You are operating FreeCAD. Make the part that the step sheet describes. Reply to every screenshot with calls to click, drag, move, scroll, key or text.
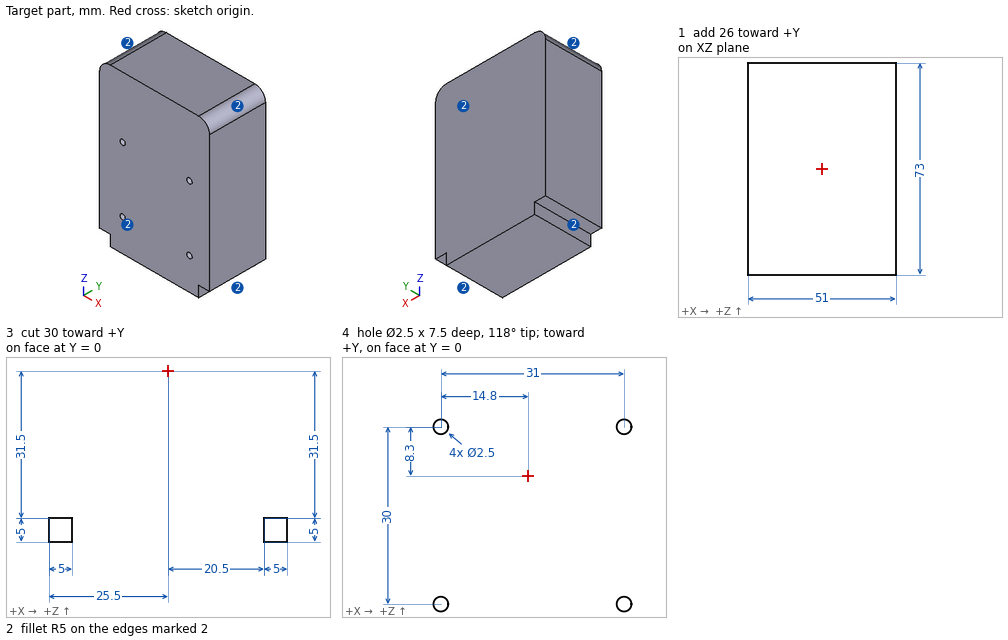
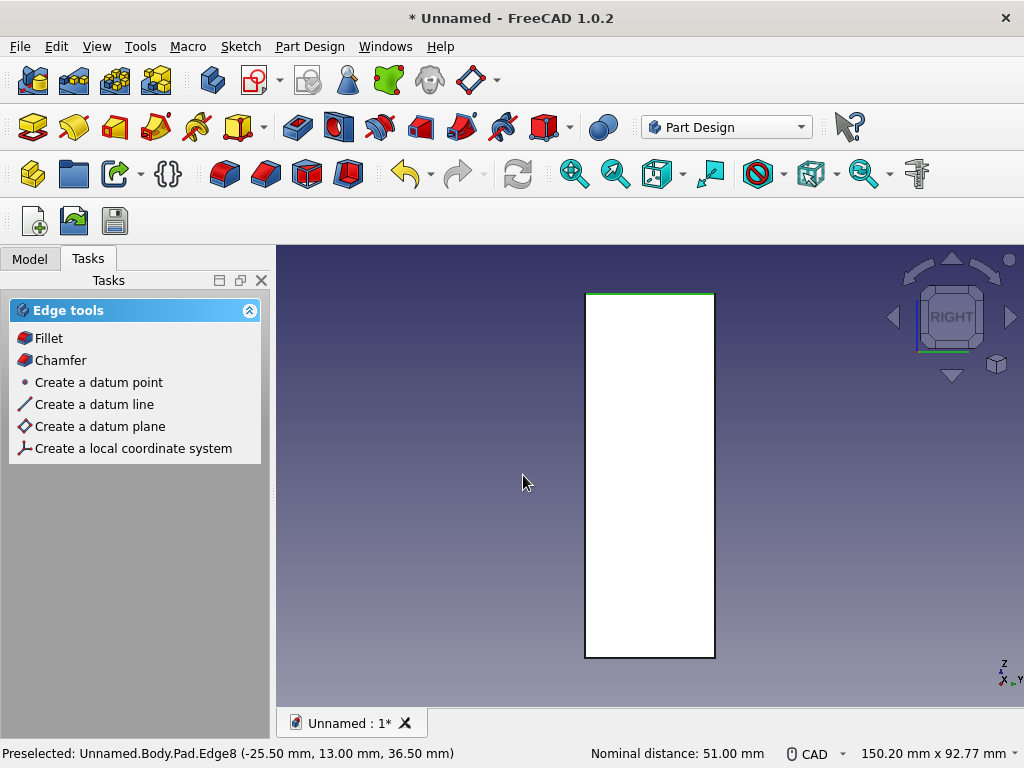
click(650, 657, ctrl)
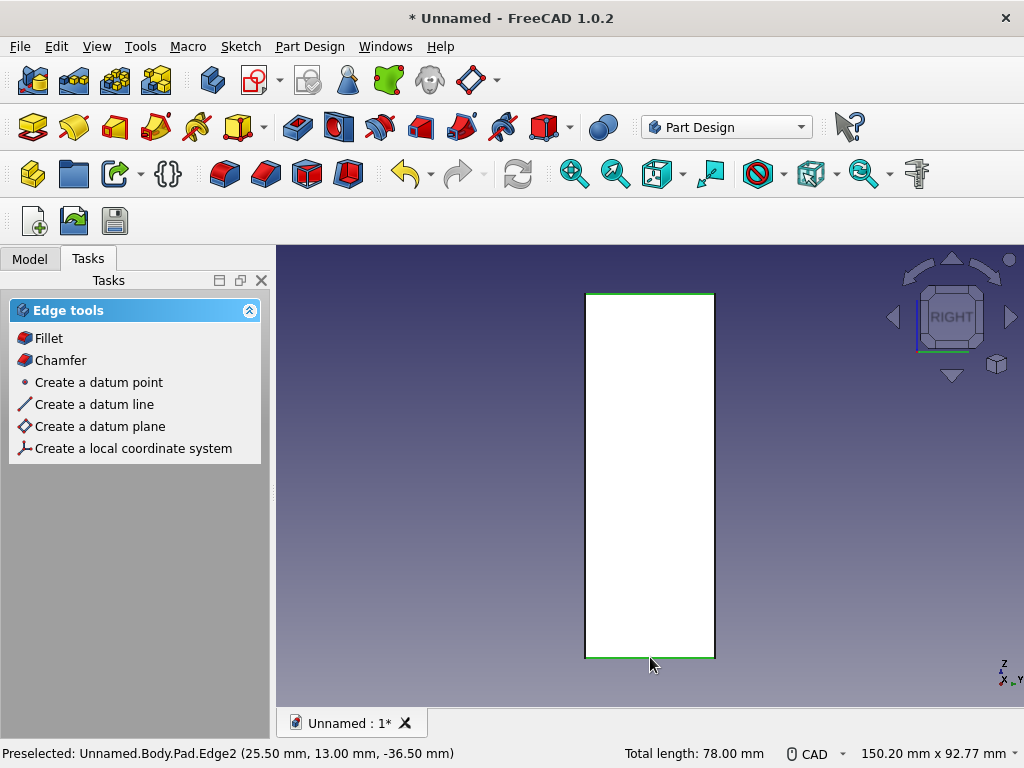
key(5)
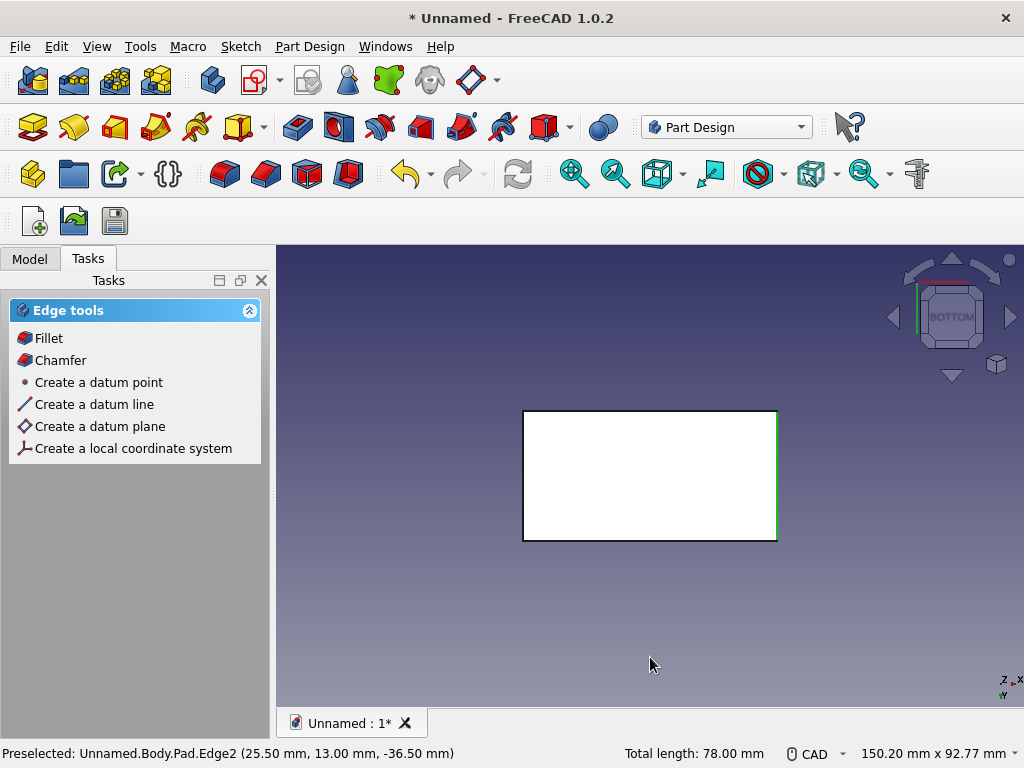
click(575, 174)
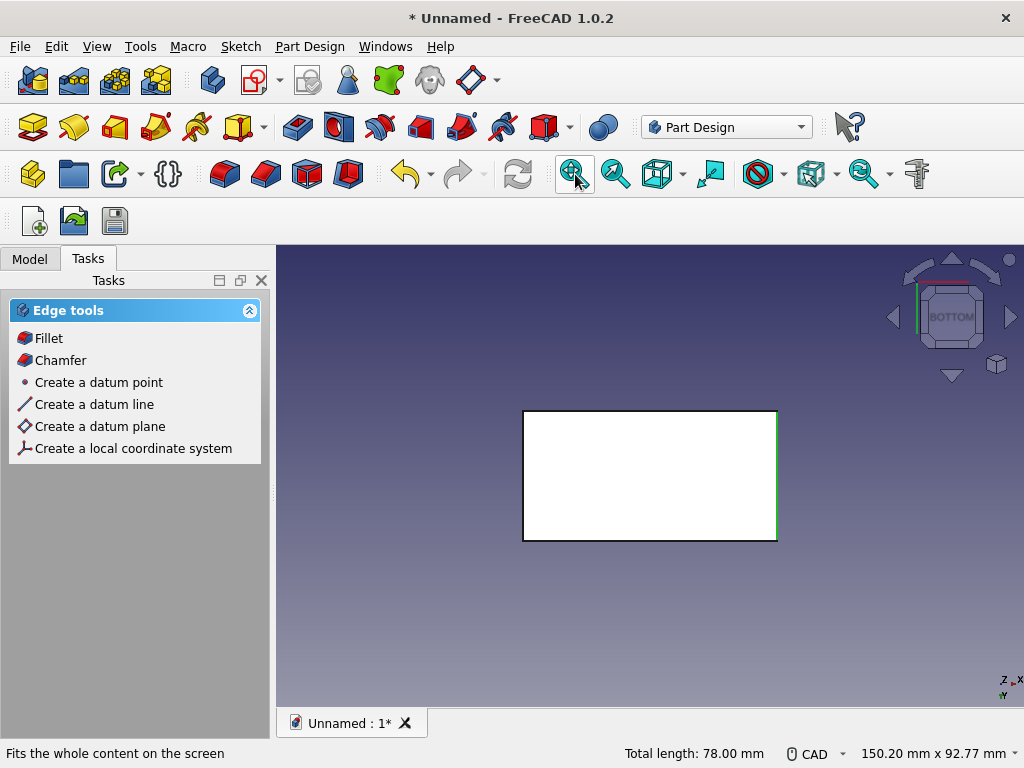
click(523, 475, ctrl)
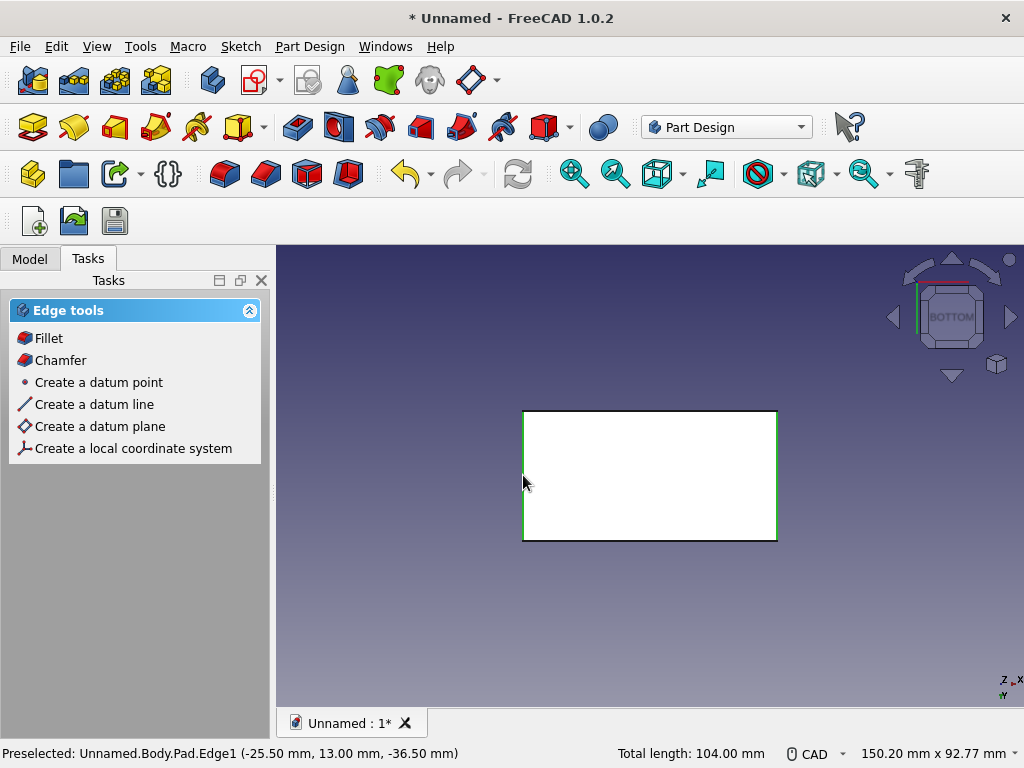
click(225, 174)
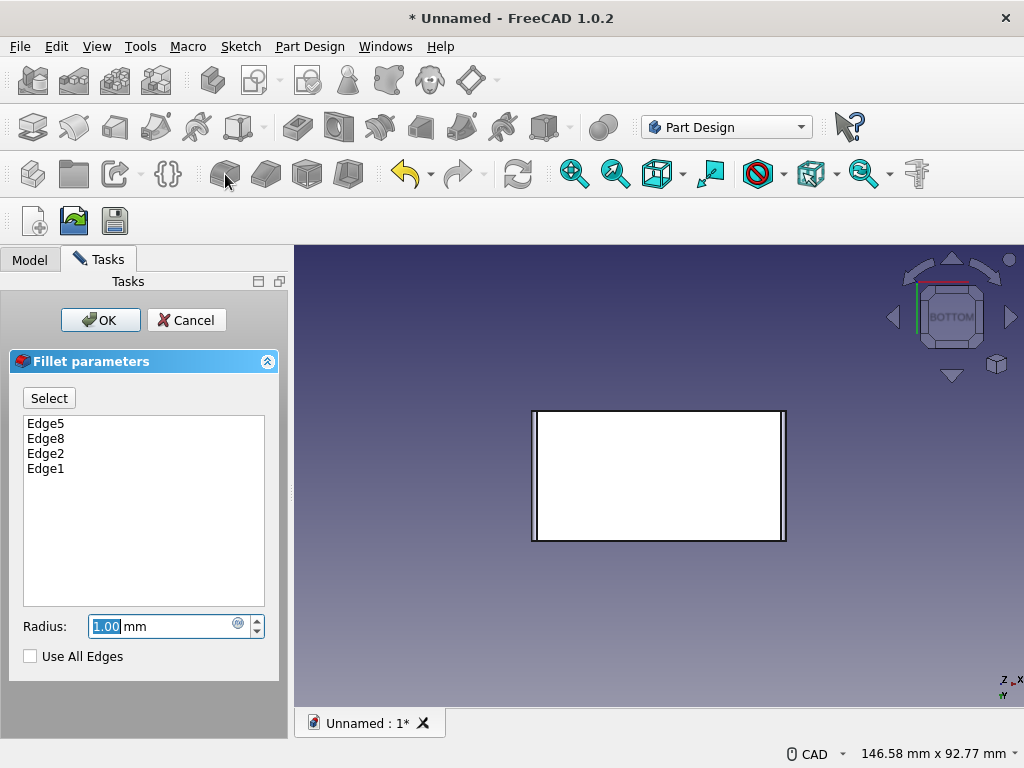
text(5)
key(Tab)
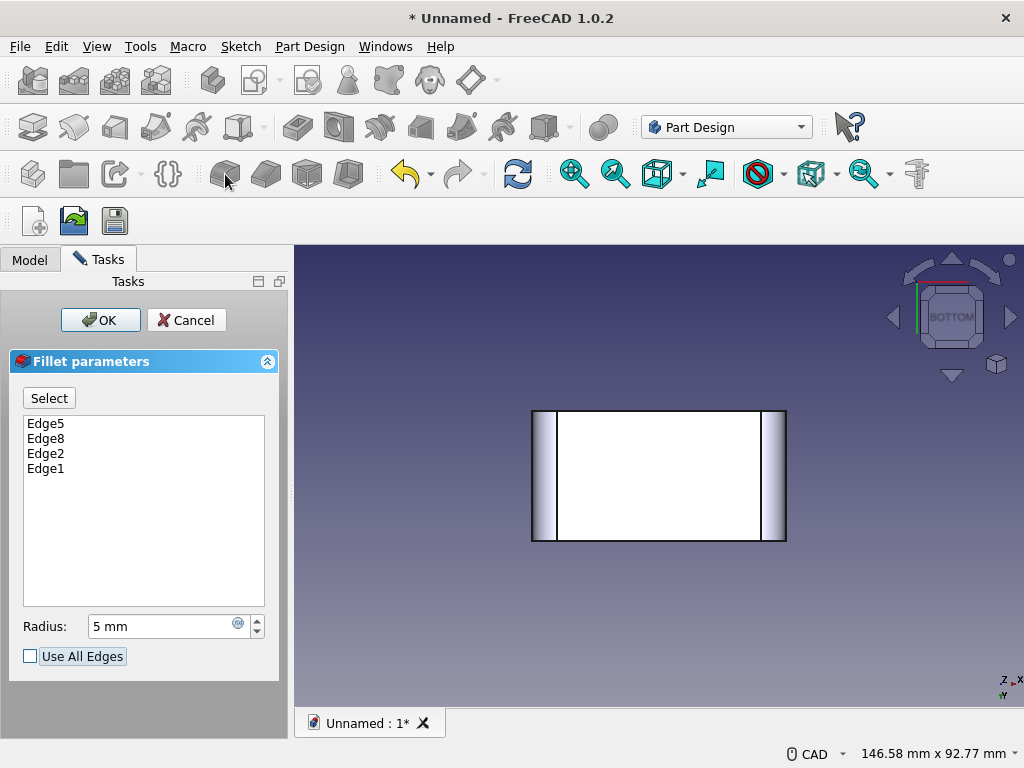
click(101, 320)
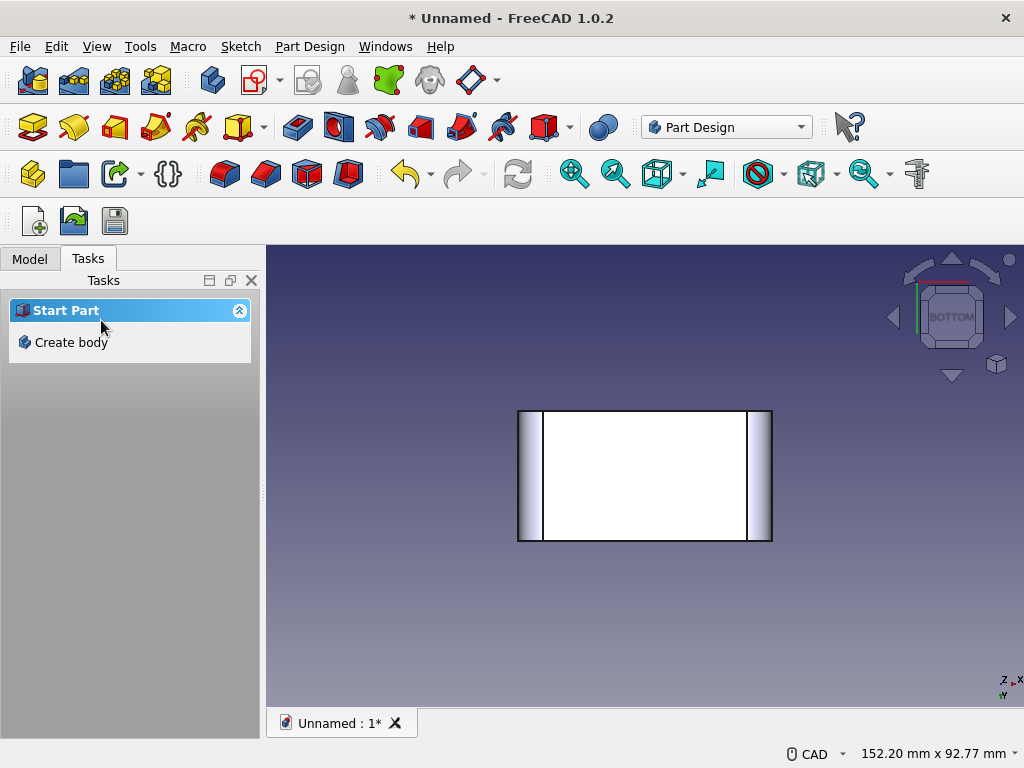
click(575, 174)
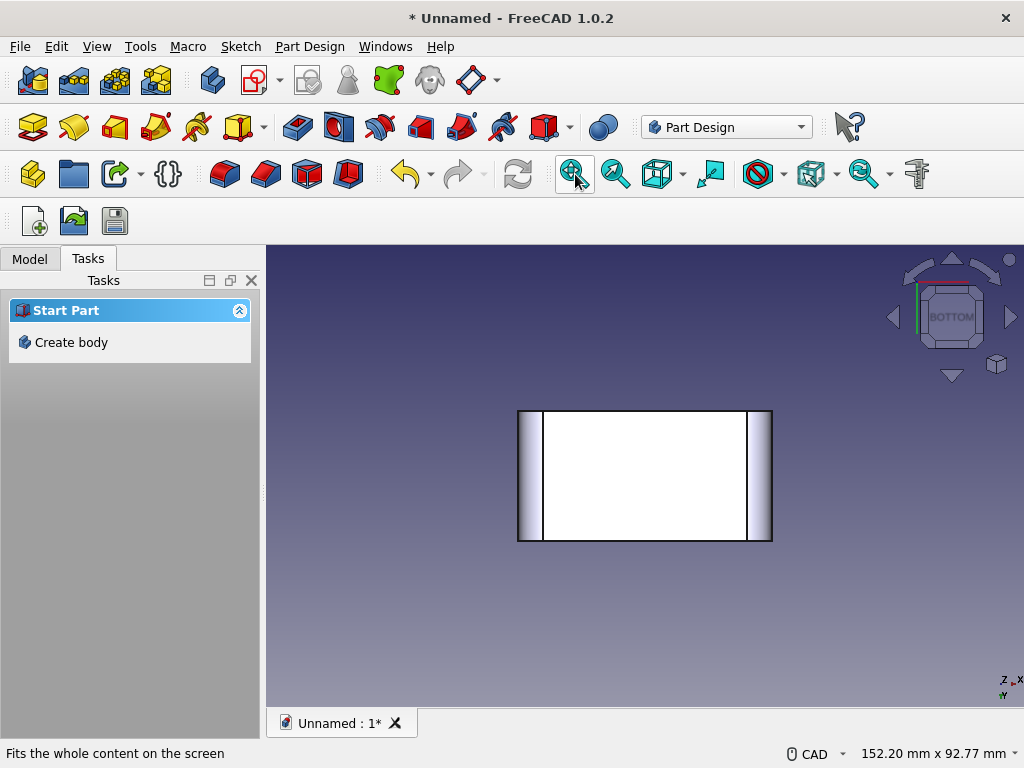
key(0)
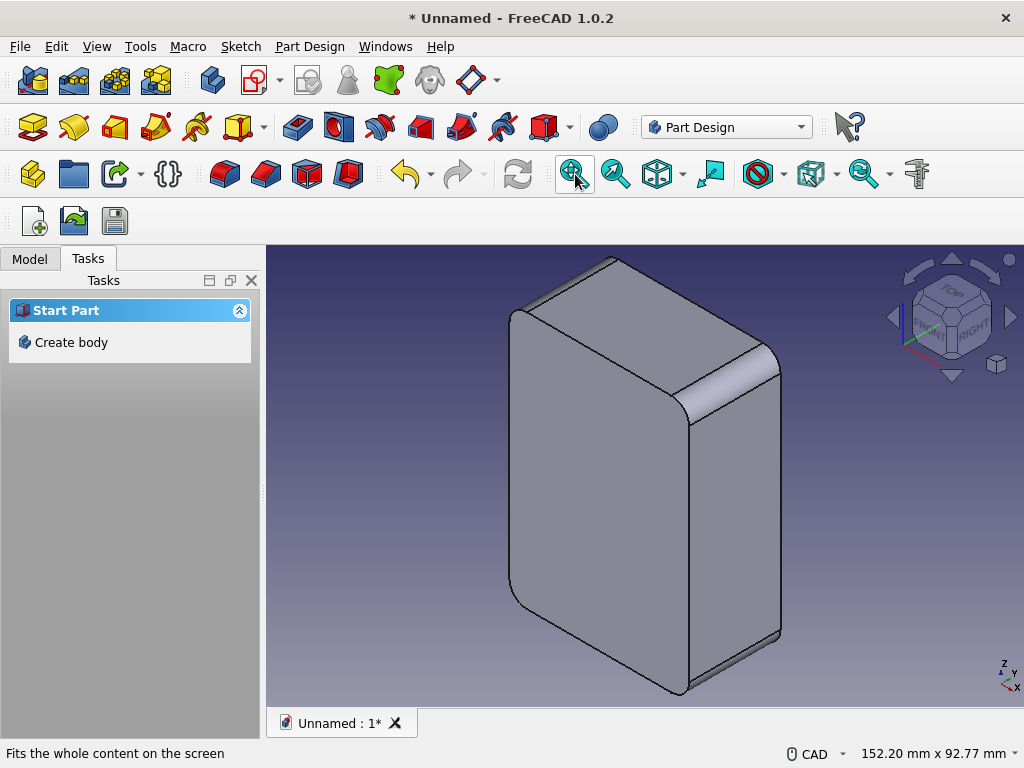
click(599, 459)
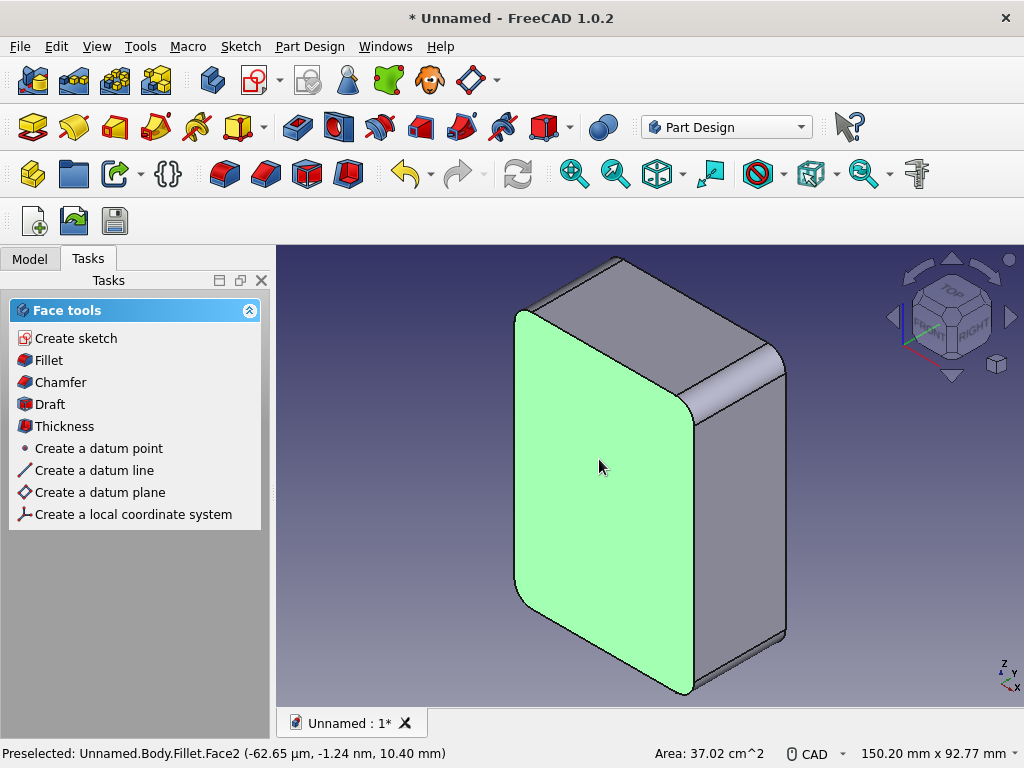
click(254, 80)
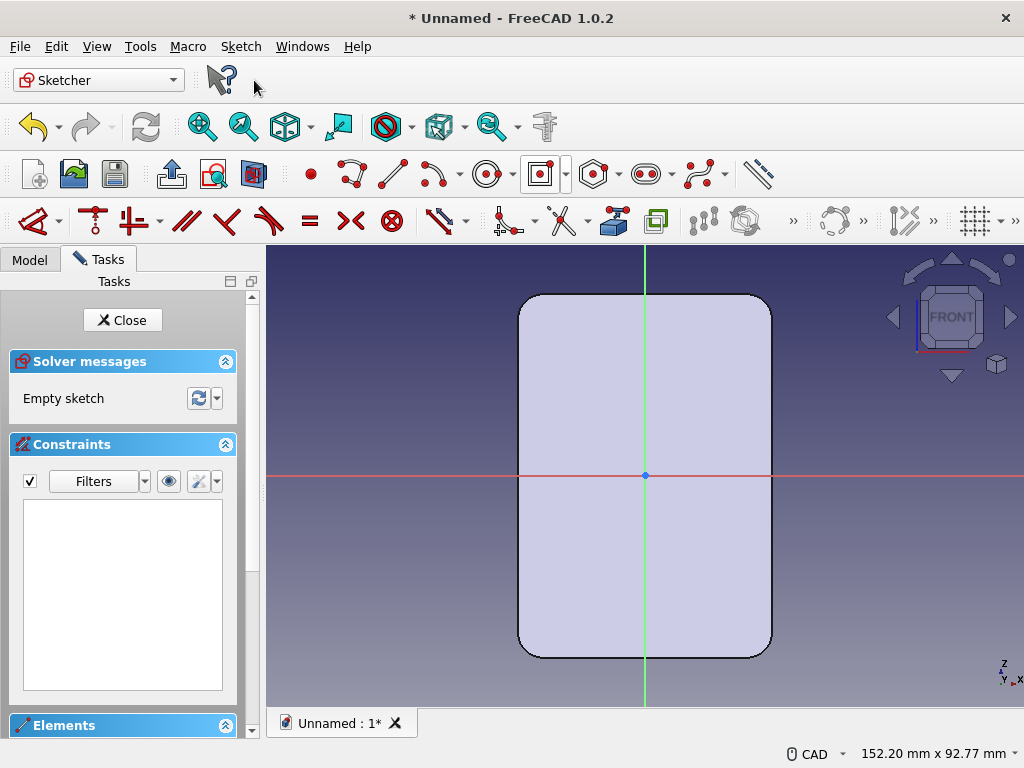
scroll(784, 679, up, 2)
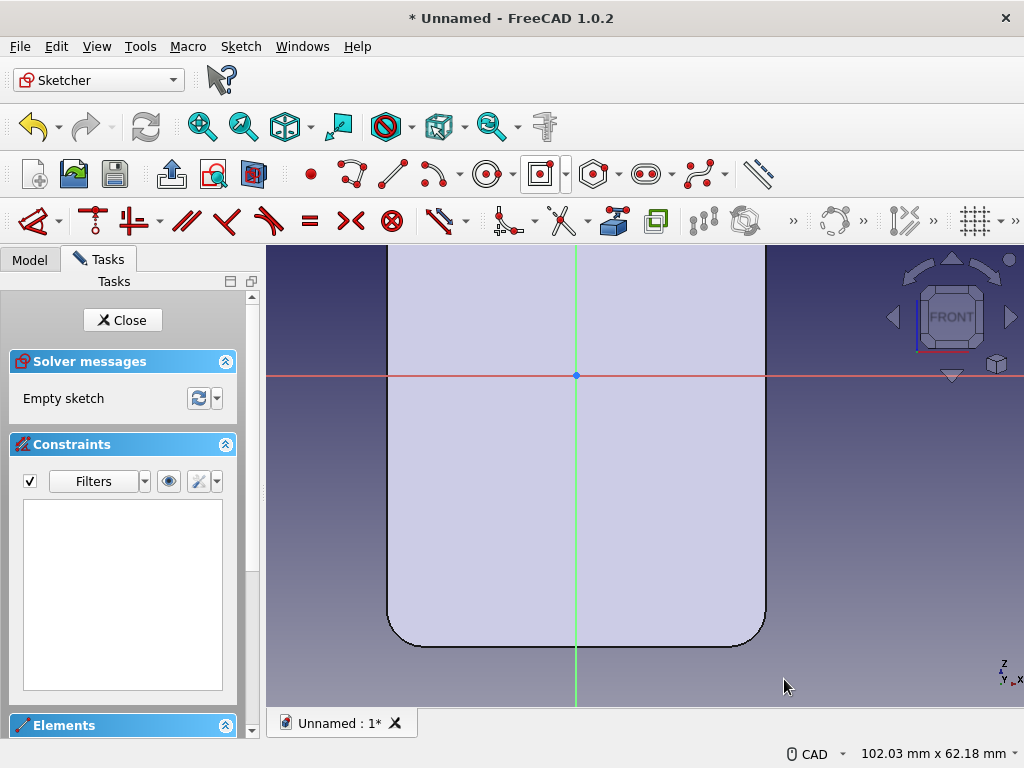
click(566, 174)